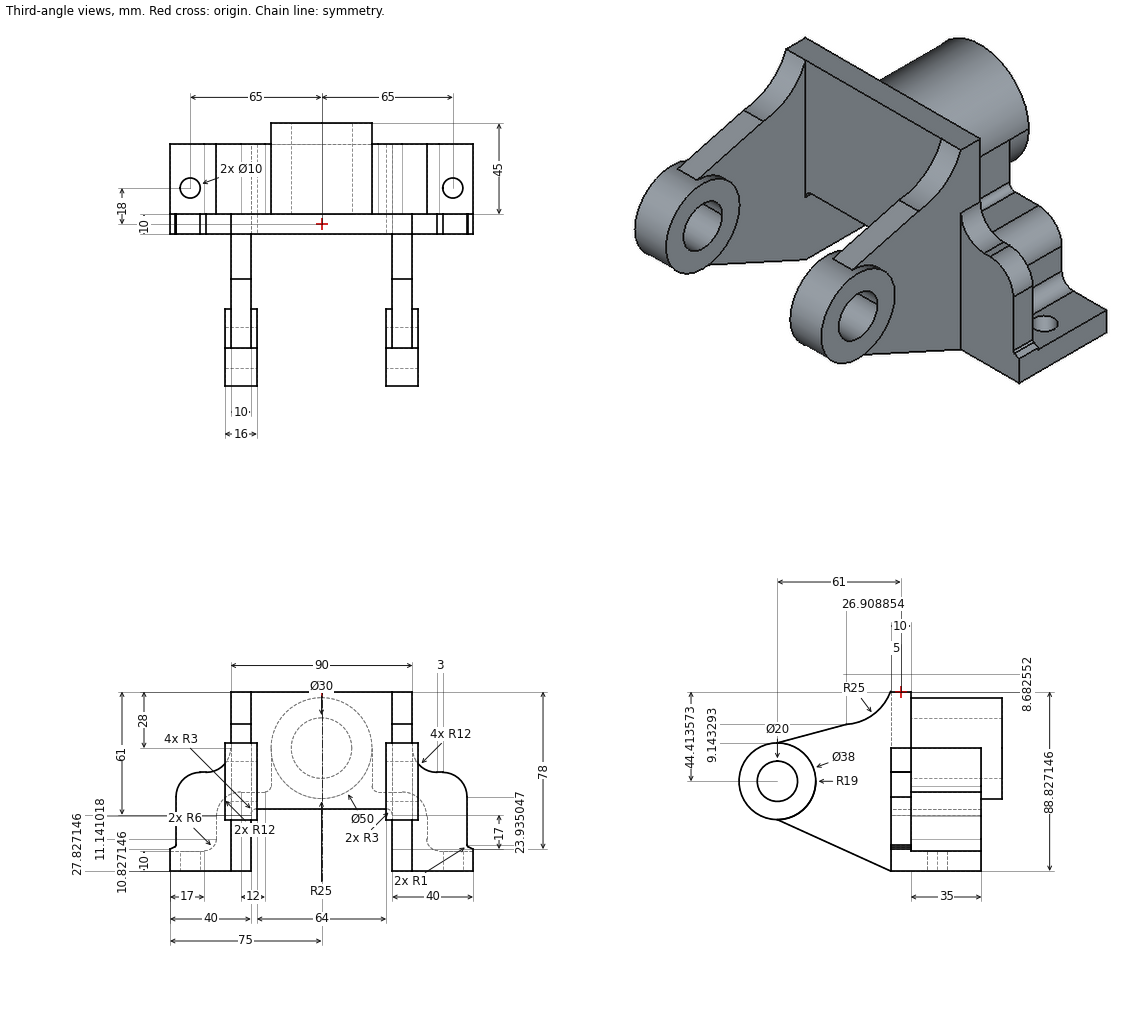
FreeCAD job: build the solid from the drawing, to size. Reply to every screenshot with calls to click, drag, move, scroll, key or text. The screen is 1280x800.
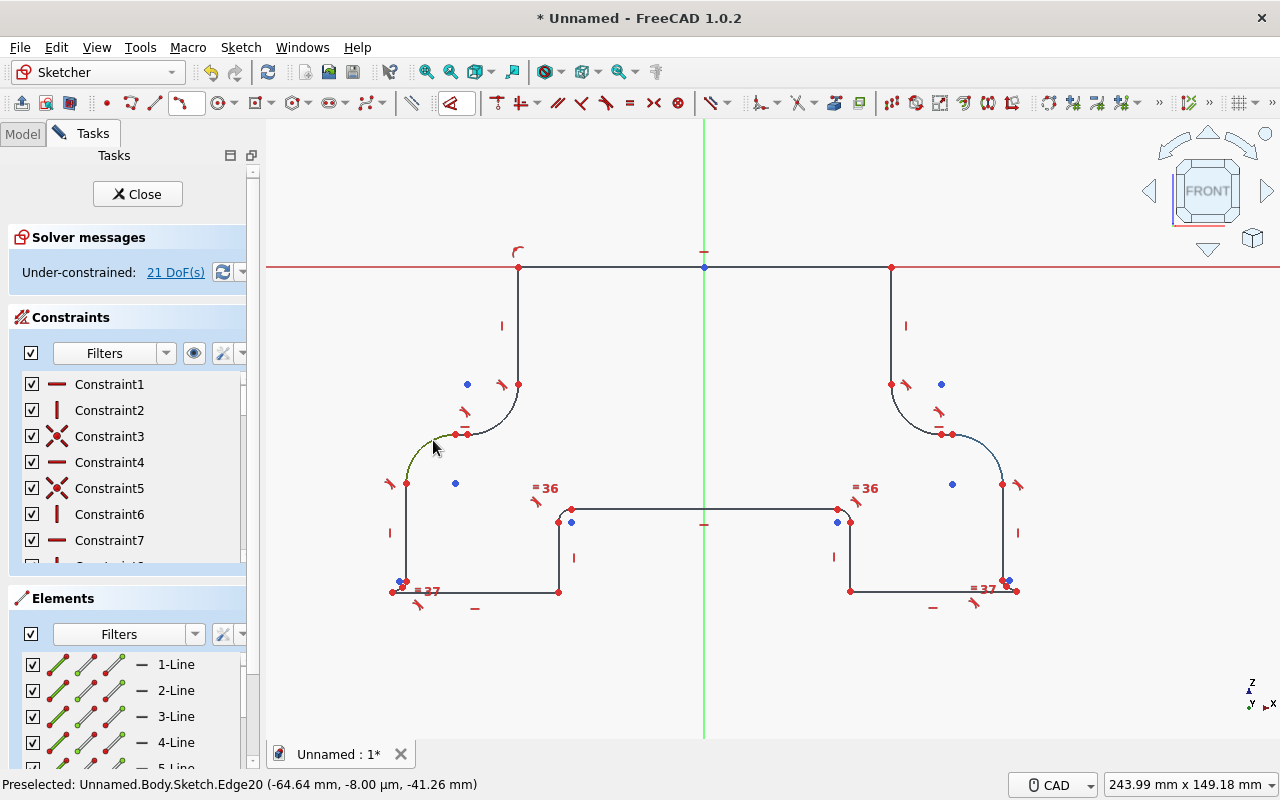
click(491, 429)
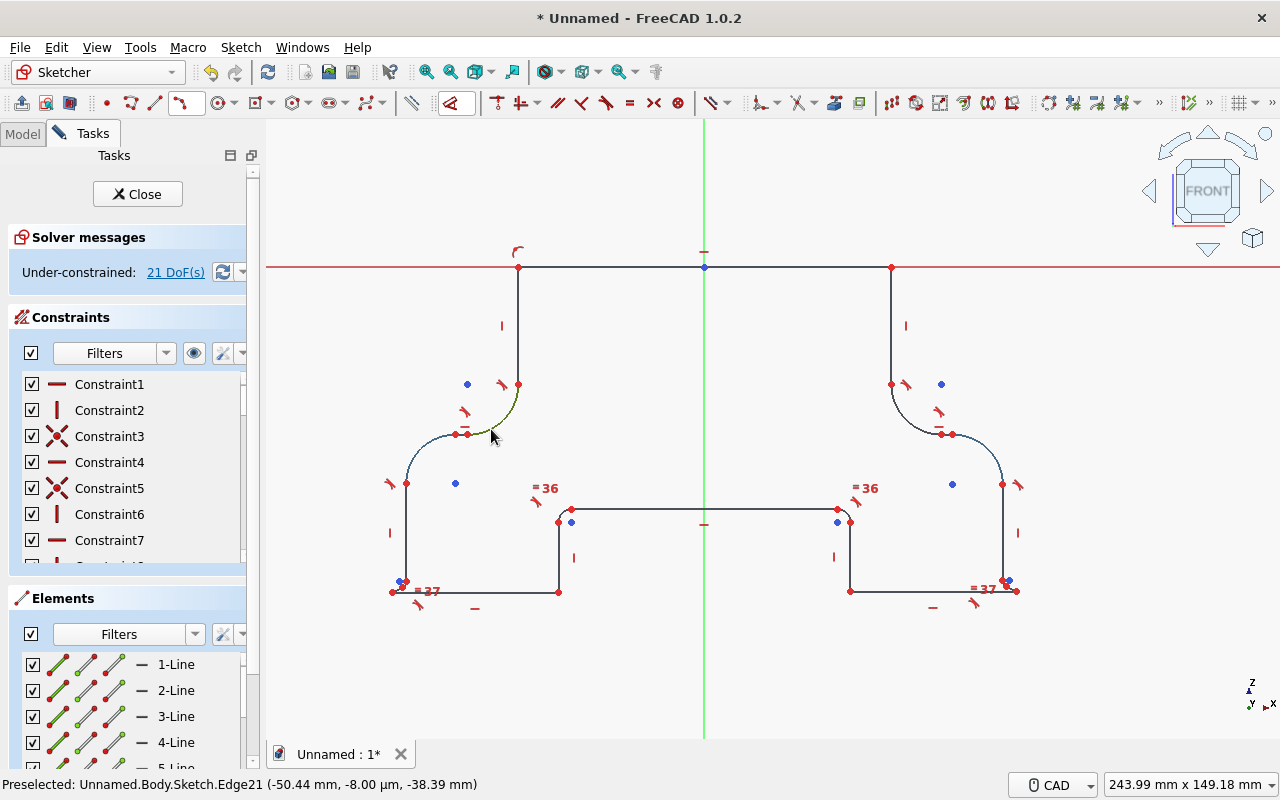
click(897, 407)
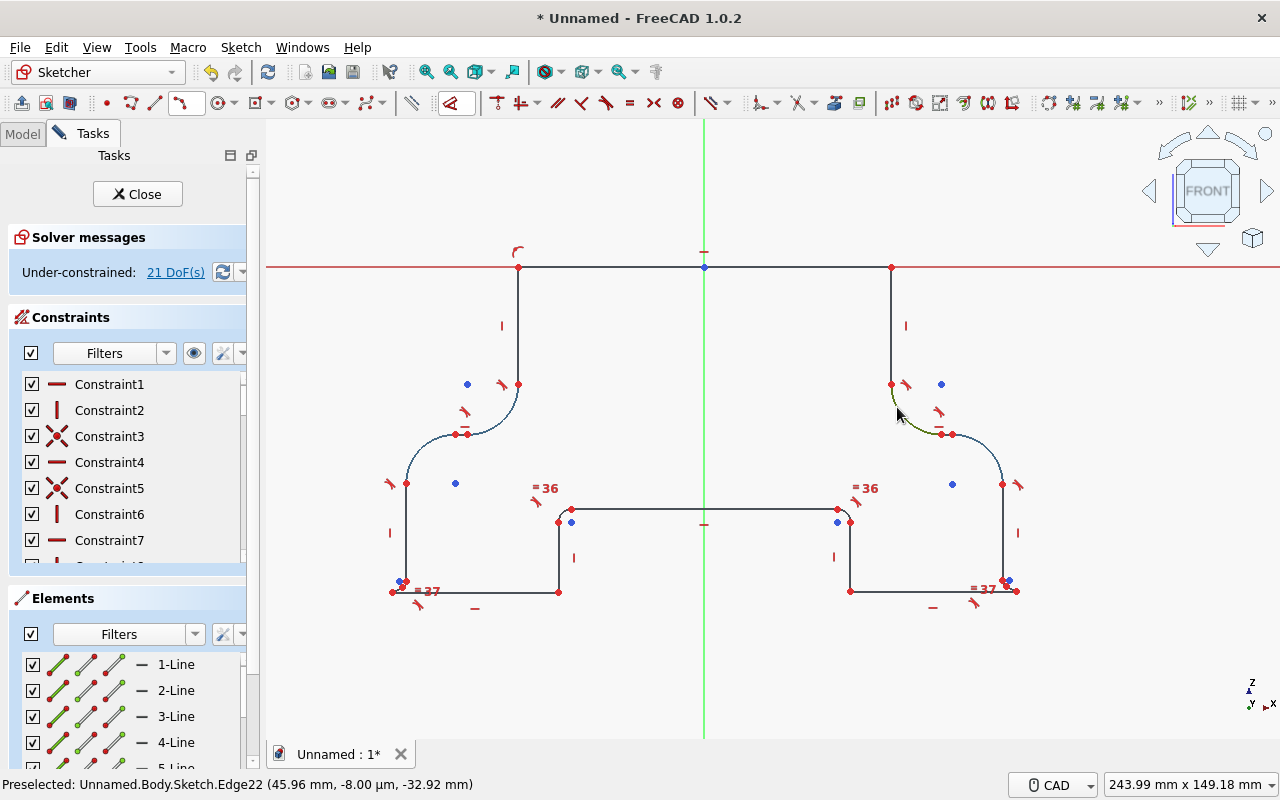
click(630, 104)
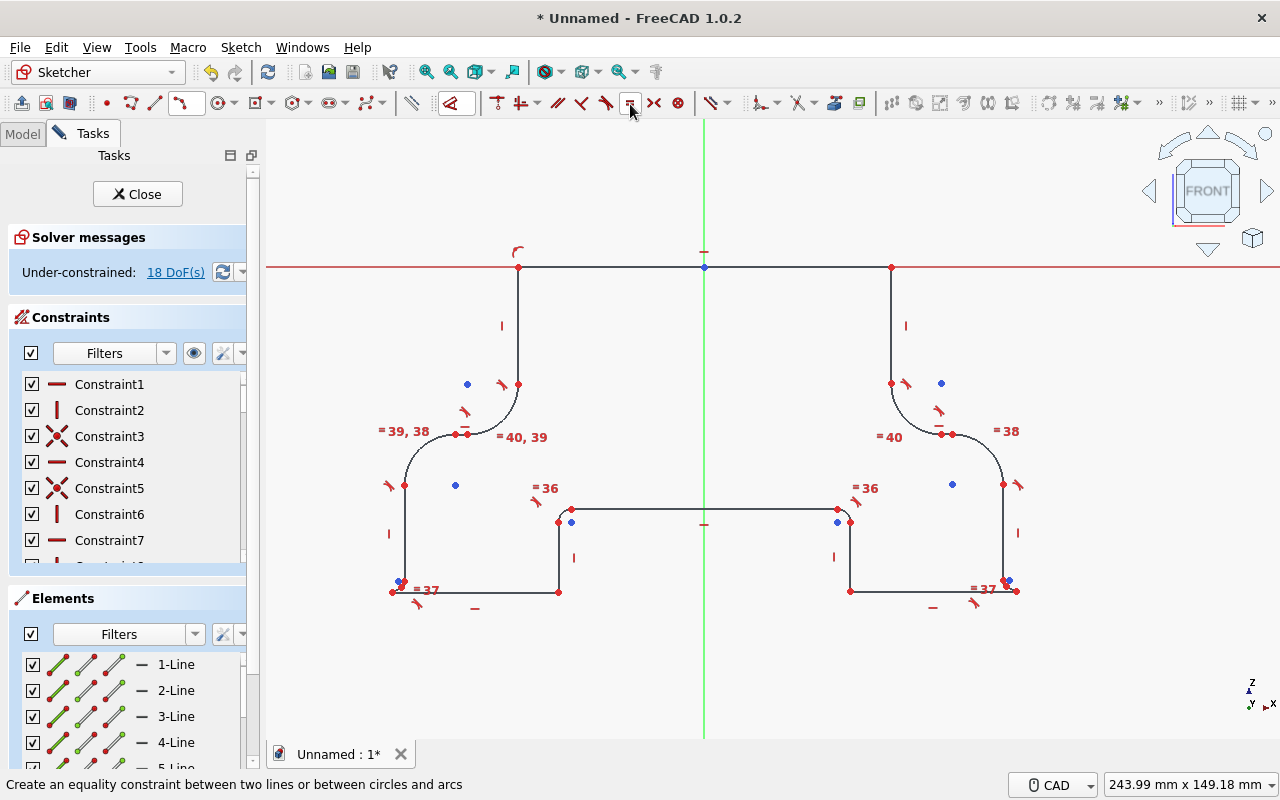
scroll(1010, 581, up, 4)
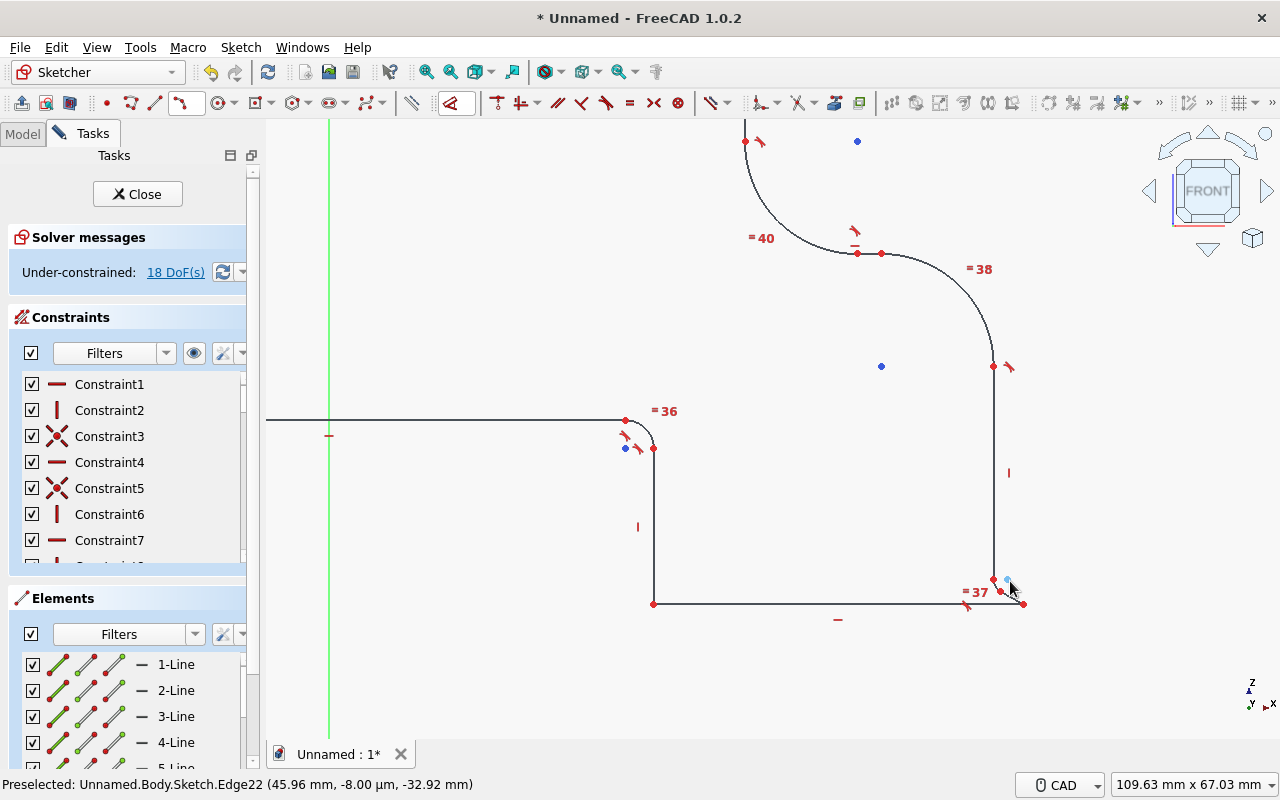
click(1008, 579)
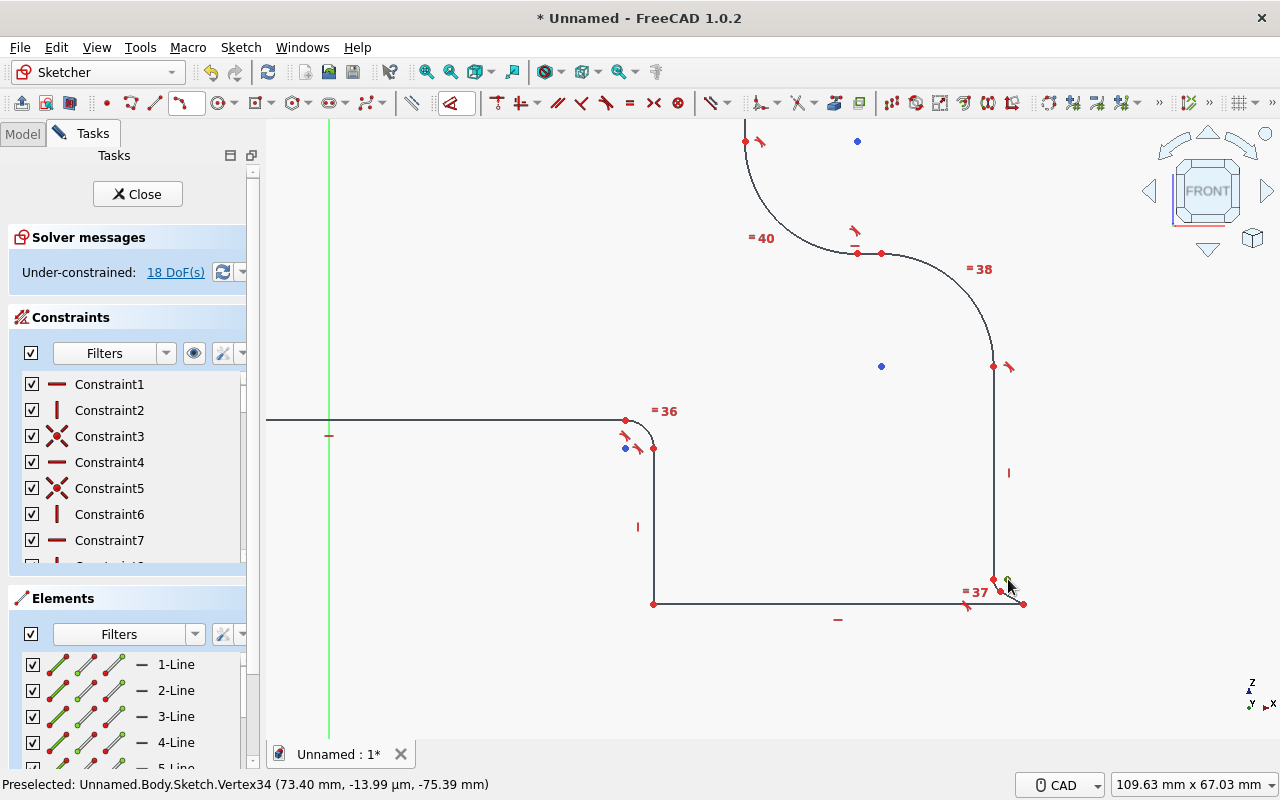
scroll(1011, 581, down, 4)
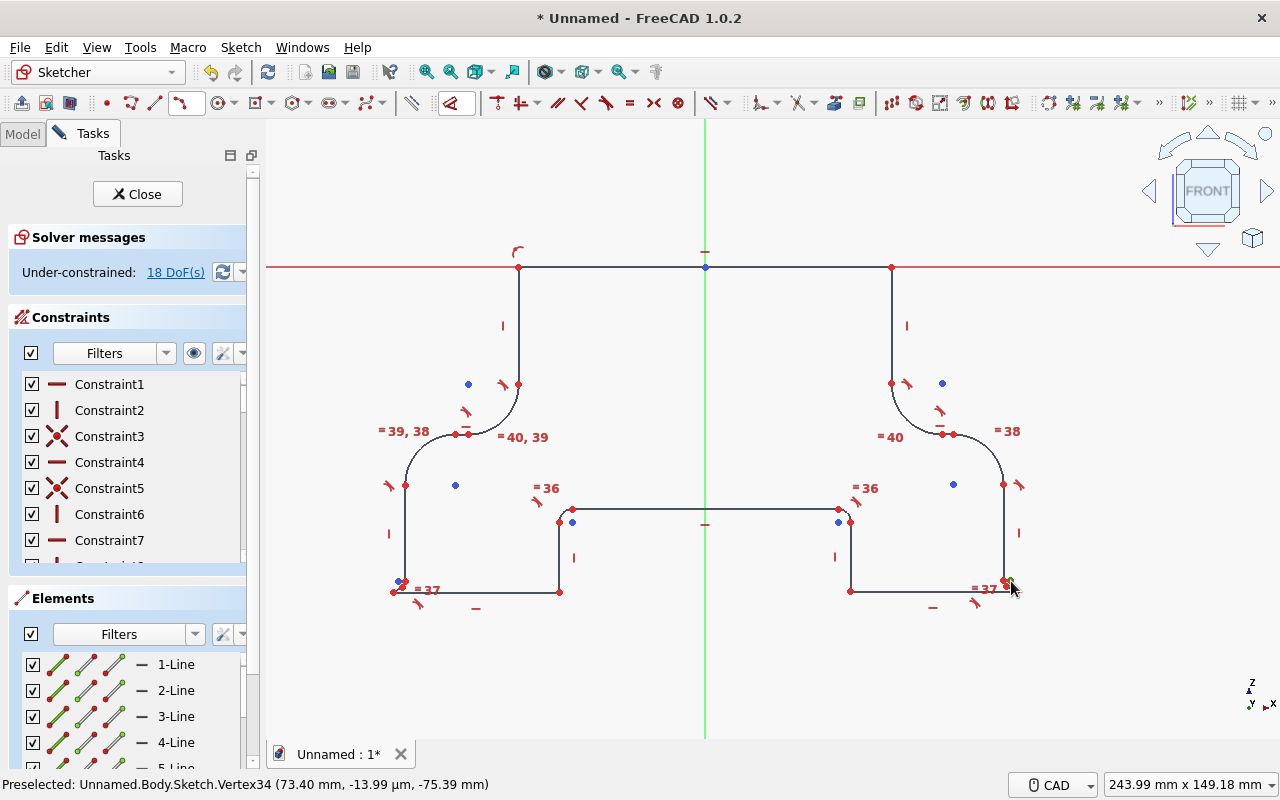
scroll(399, 582, up, 4)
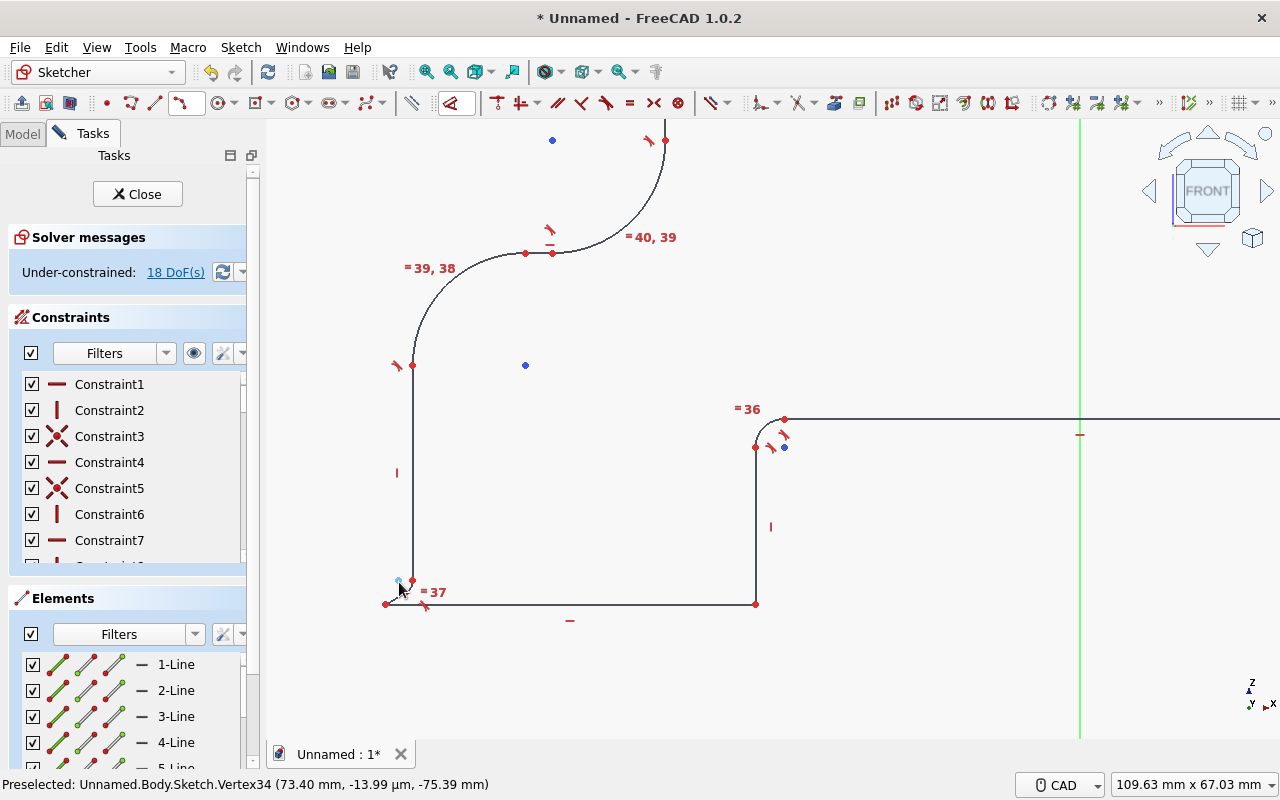
click(399, 581)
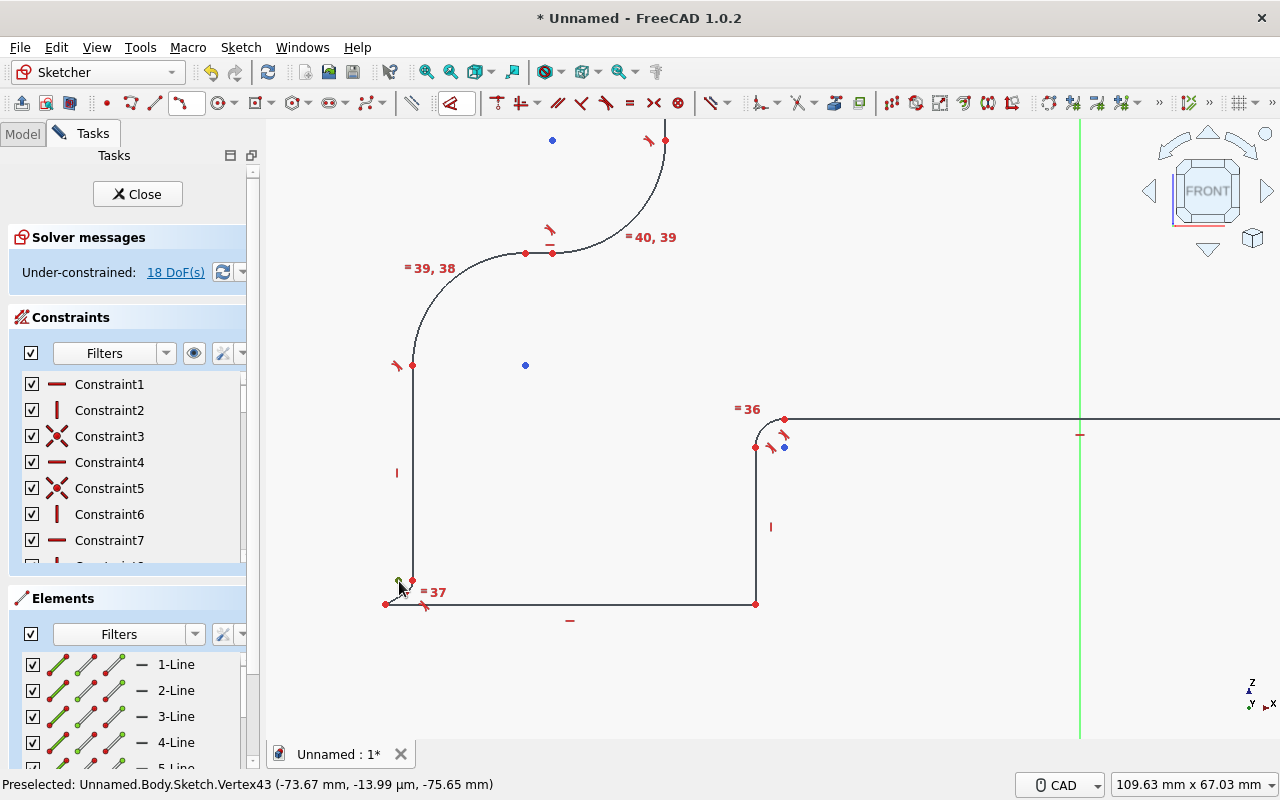
click(1080, 671)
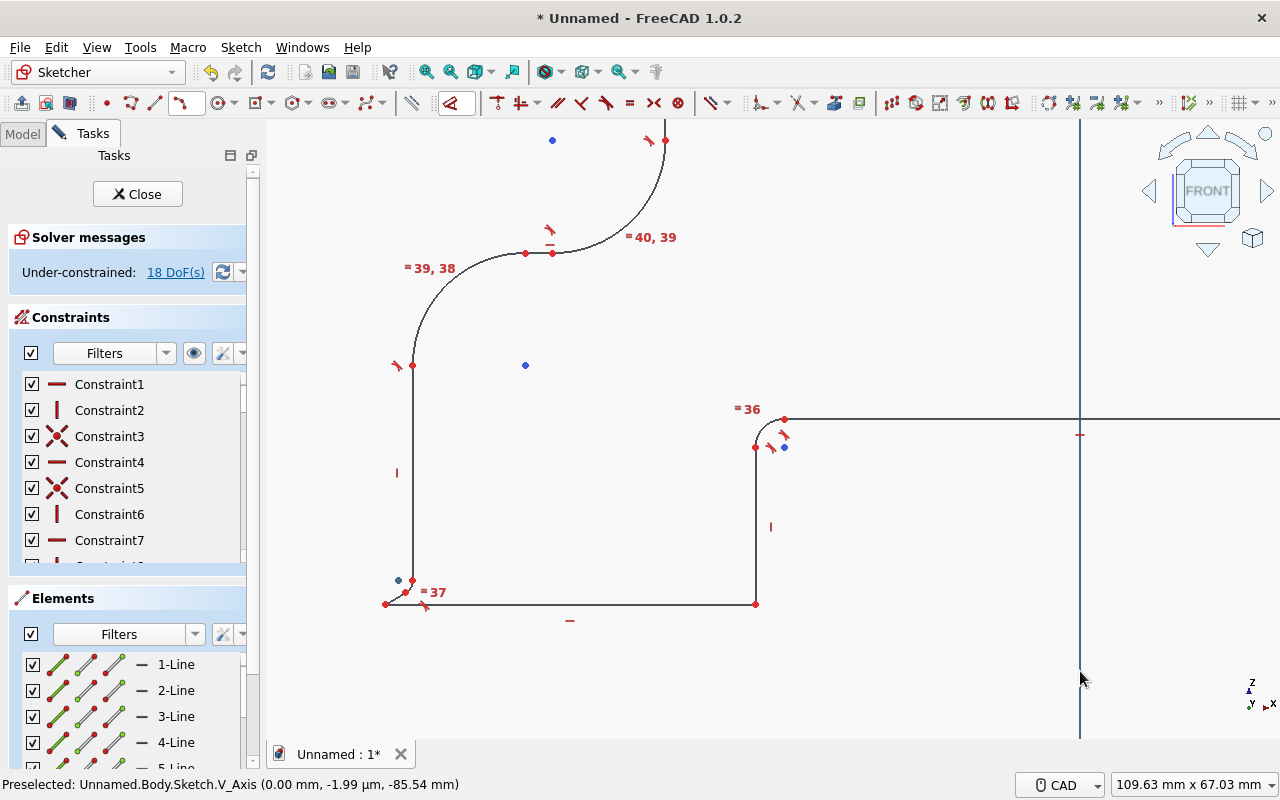
key(s)